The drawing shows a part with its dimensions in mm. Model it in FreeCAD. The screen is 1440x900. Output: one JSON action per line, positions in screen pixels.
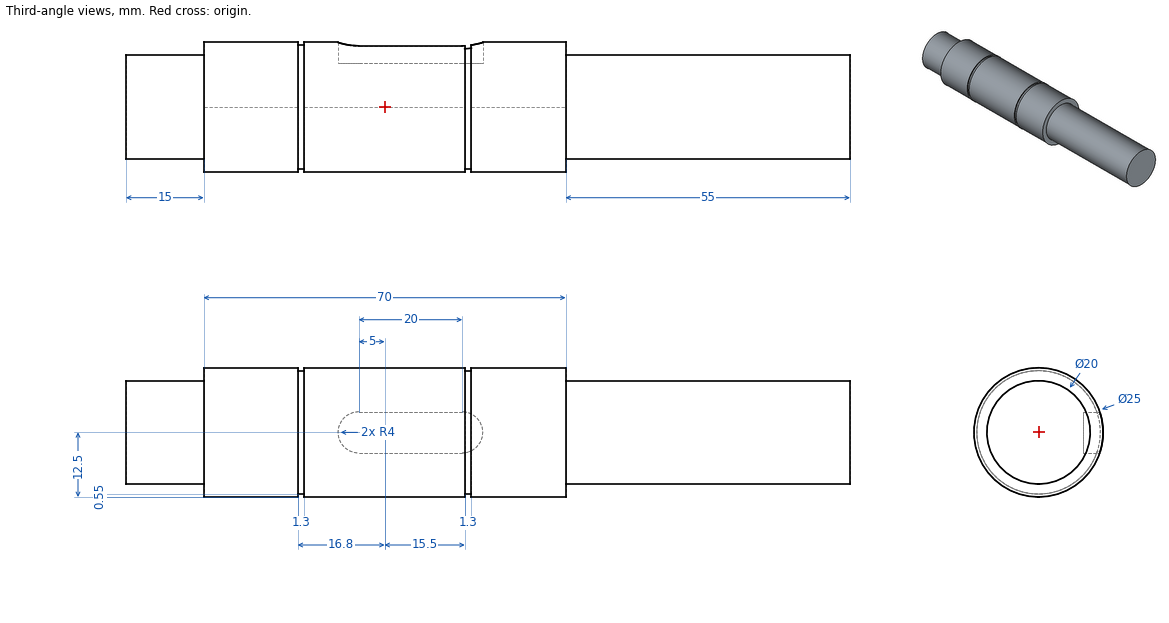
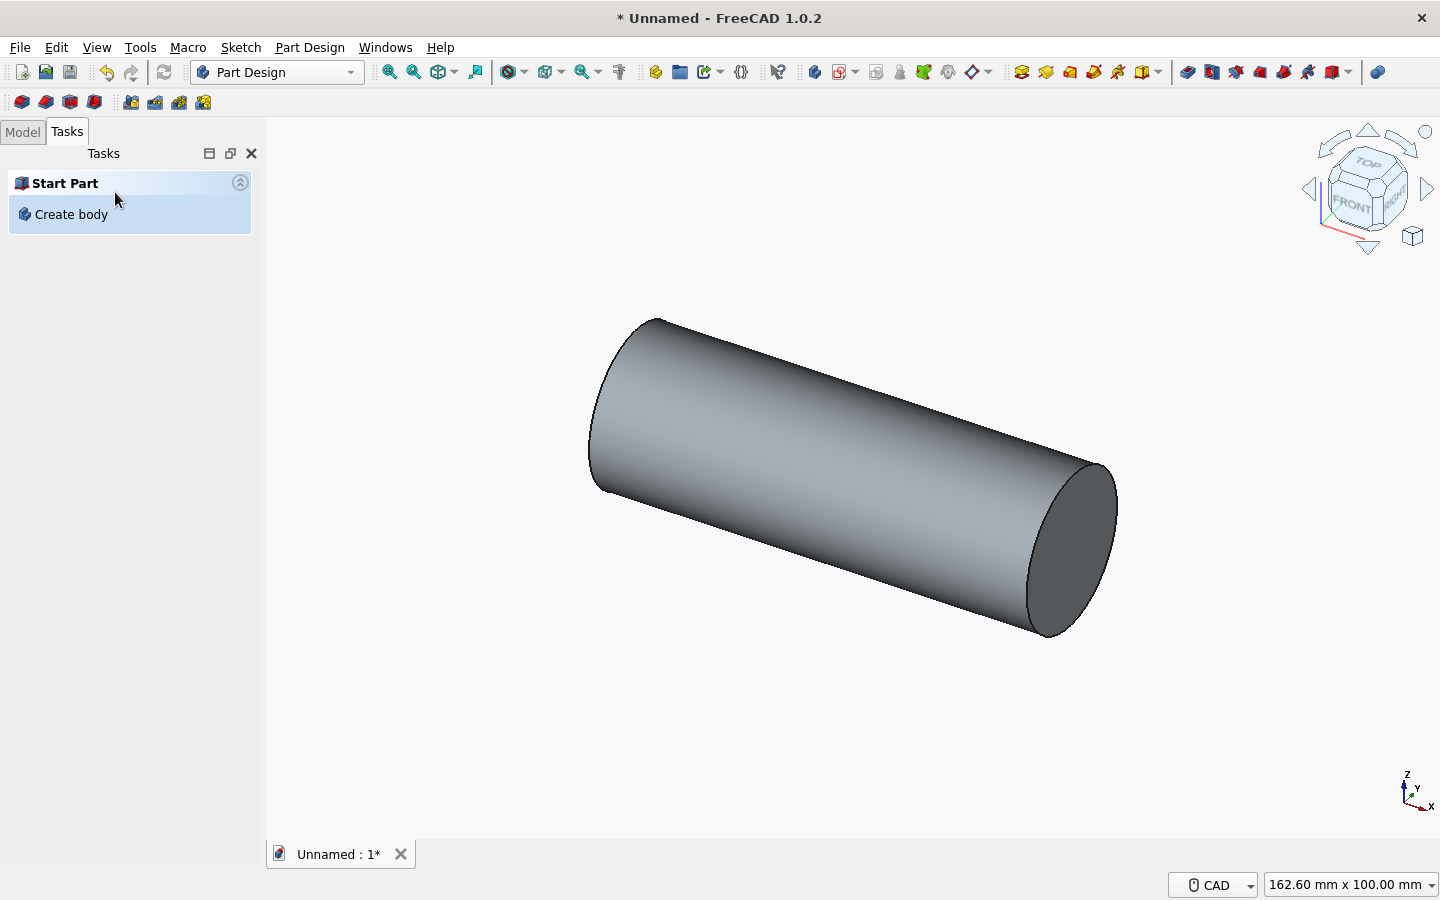
{"action": "left_click", "coordinate": [1072, 549]}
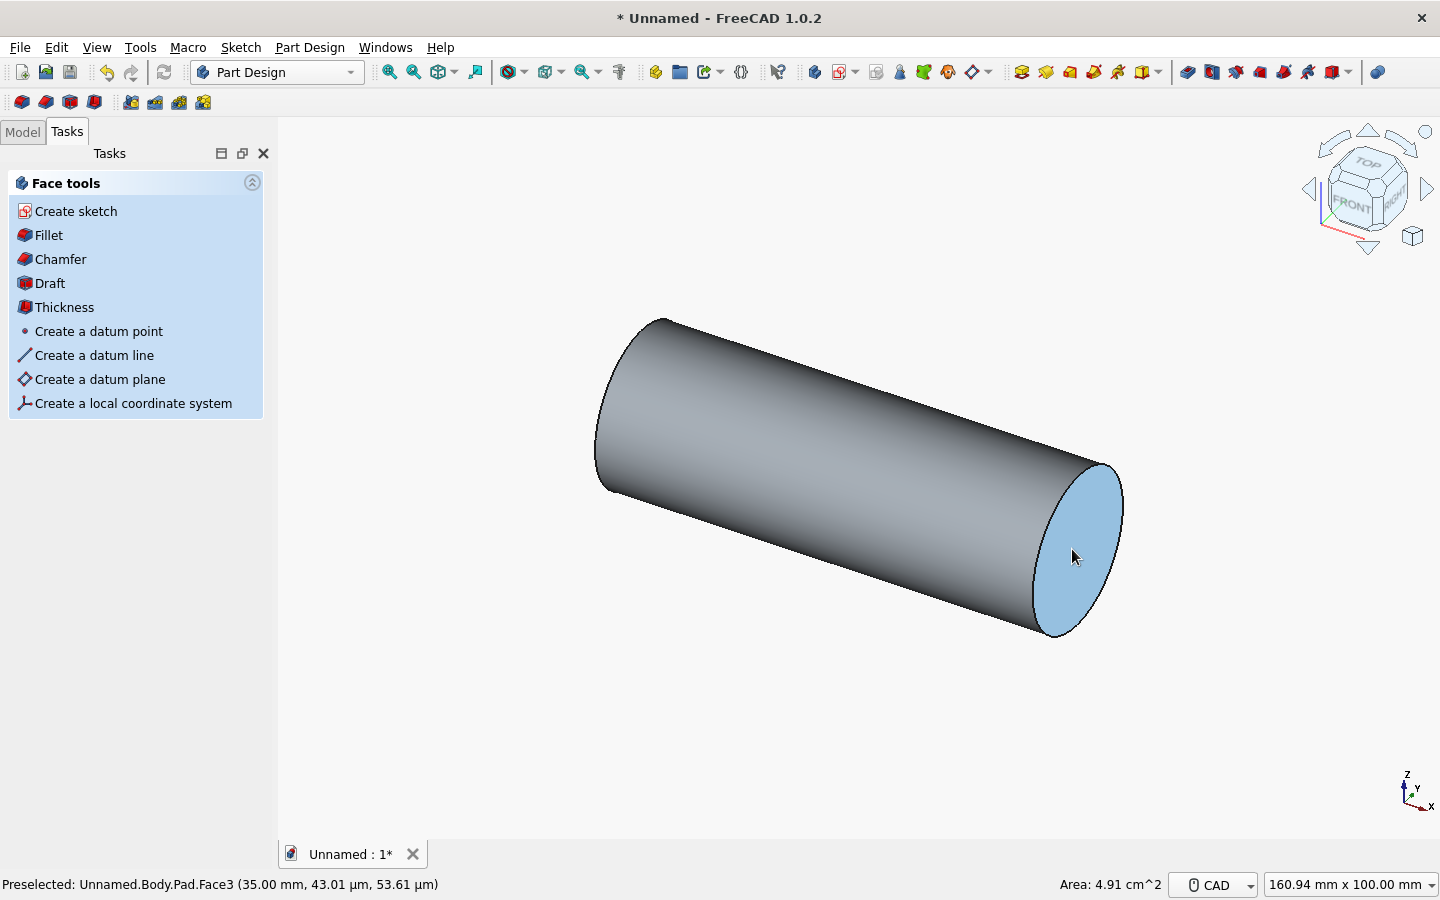
{"action": "left_click", "coordinate": [840, 72]}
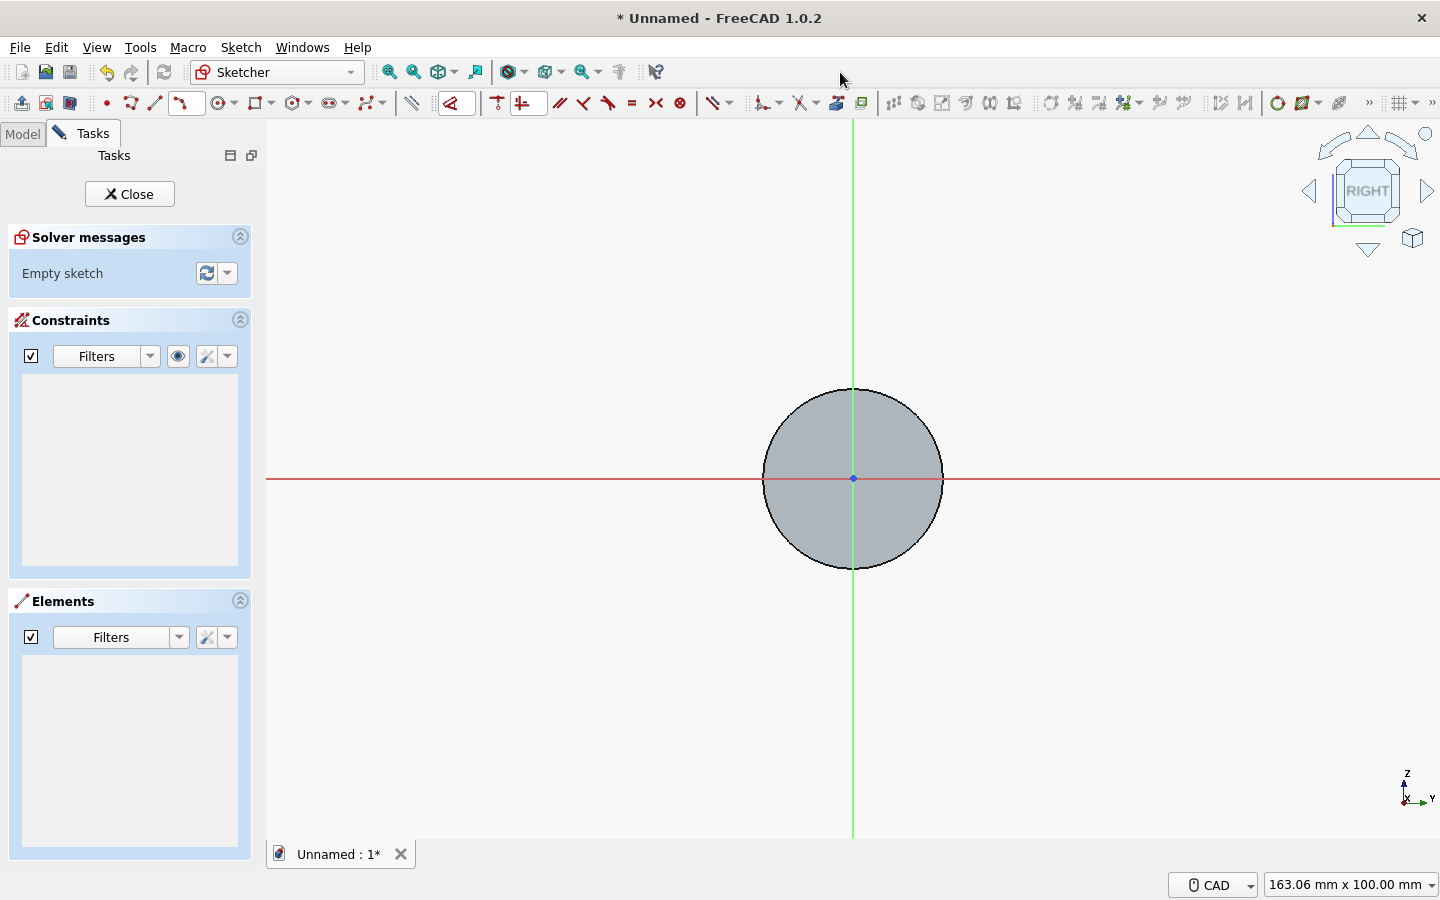
{"action": "scroll", "coordinate": [883, 479], "scroll_direction": "up", "scroll_amount": 6}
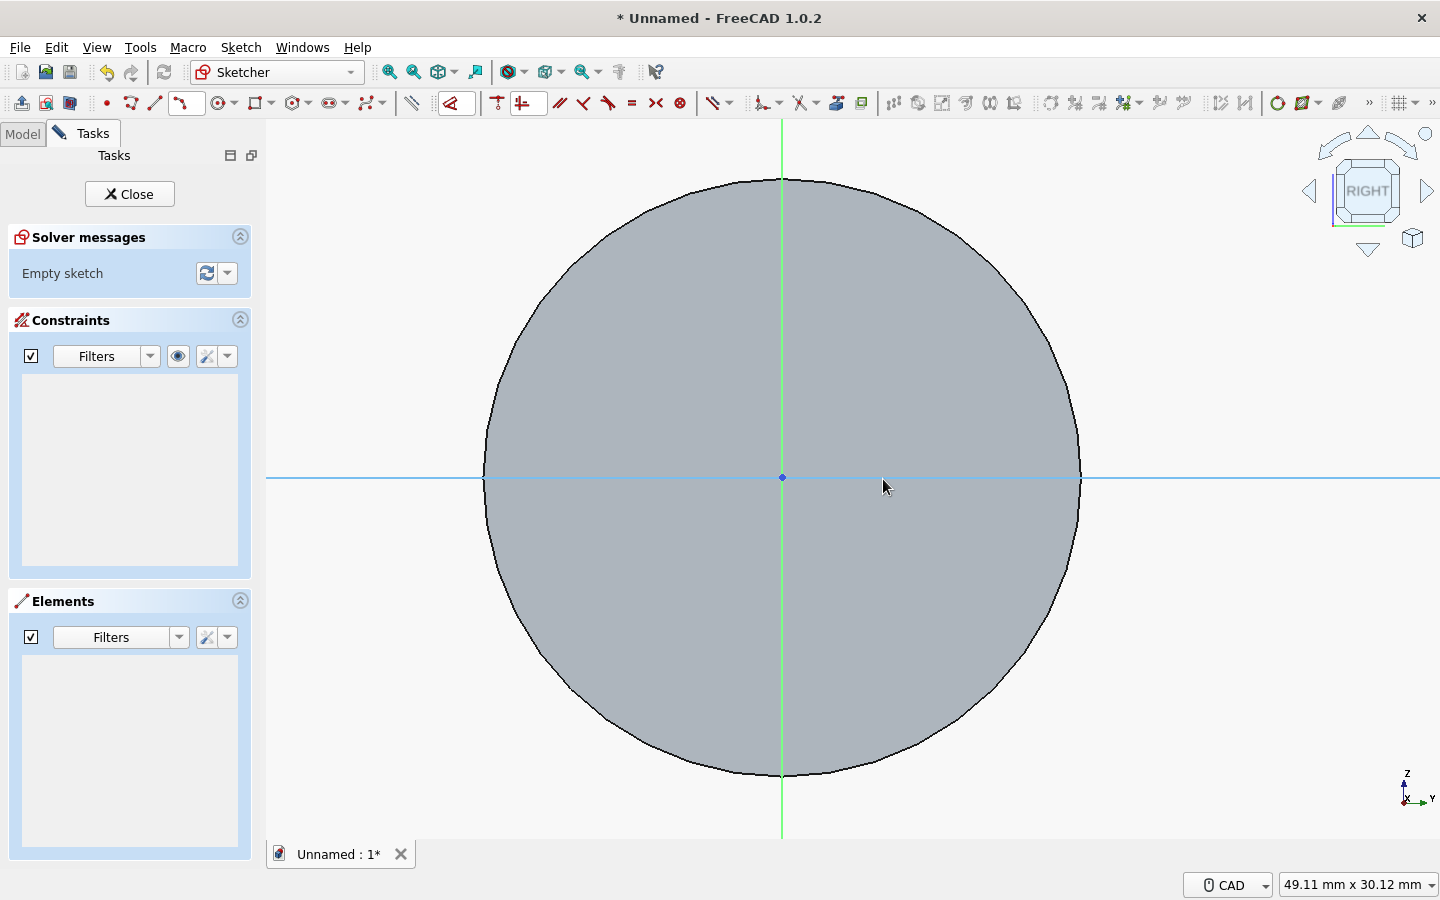
{"action": "left_click", "coordinate": [218, 104]}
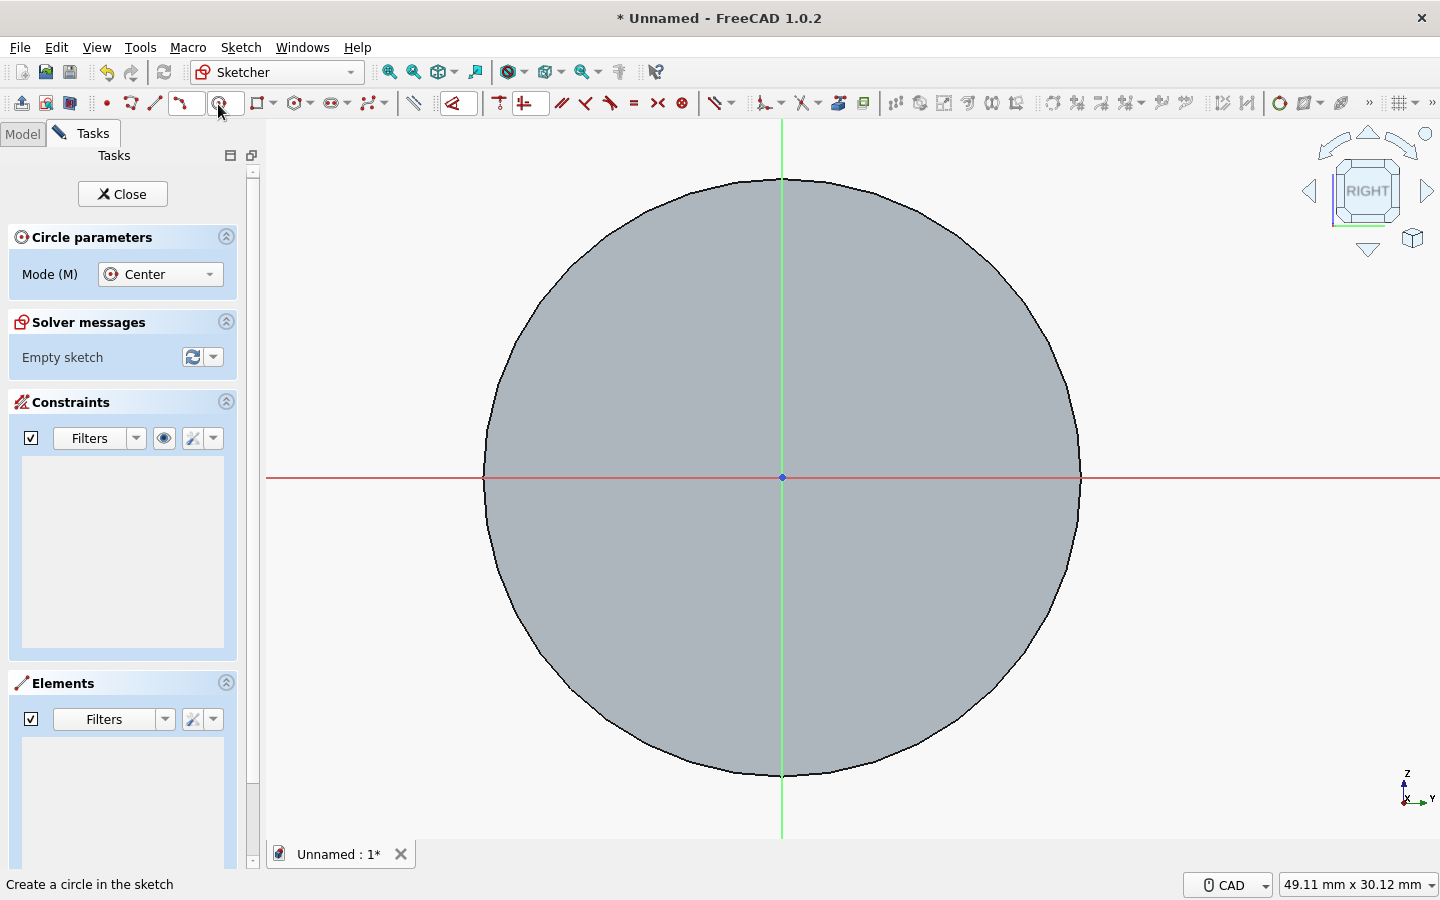
{"action": "left_click", "coordinate": [782, 478]}
{"action": "left_click", "coordinate": [951, 309]}
{"action": "key", "text": "Escape"}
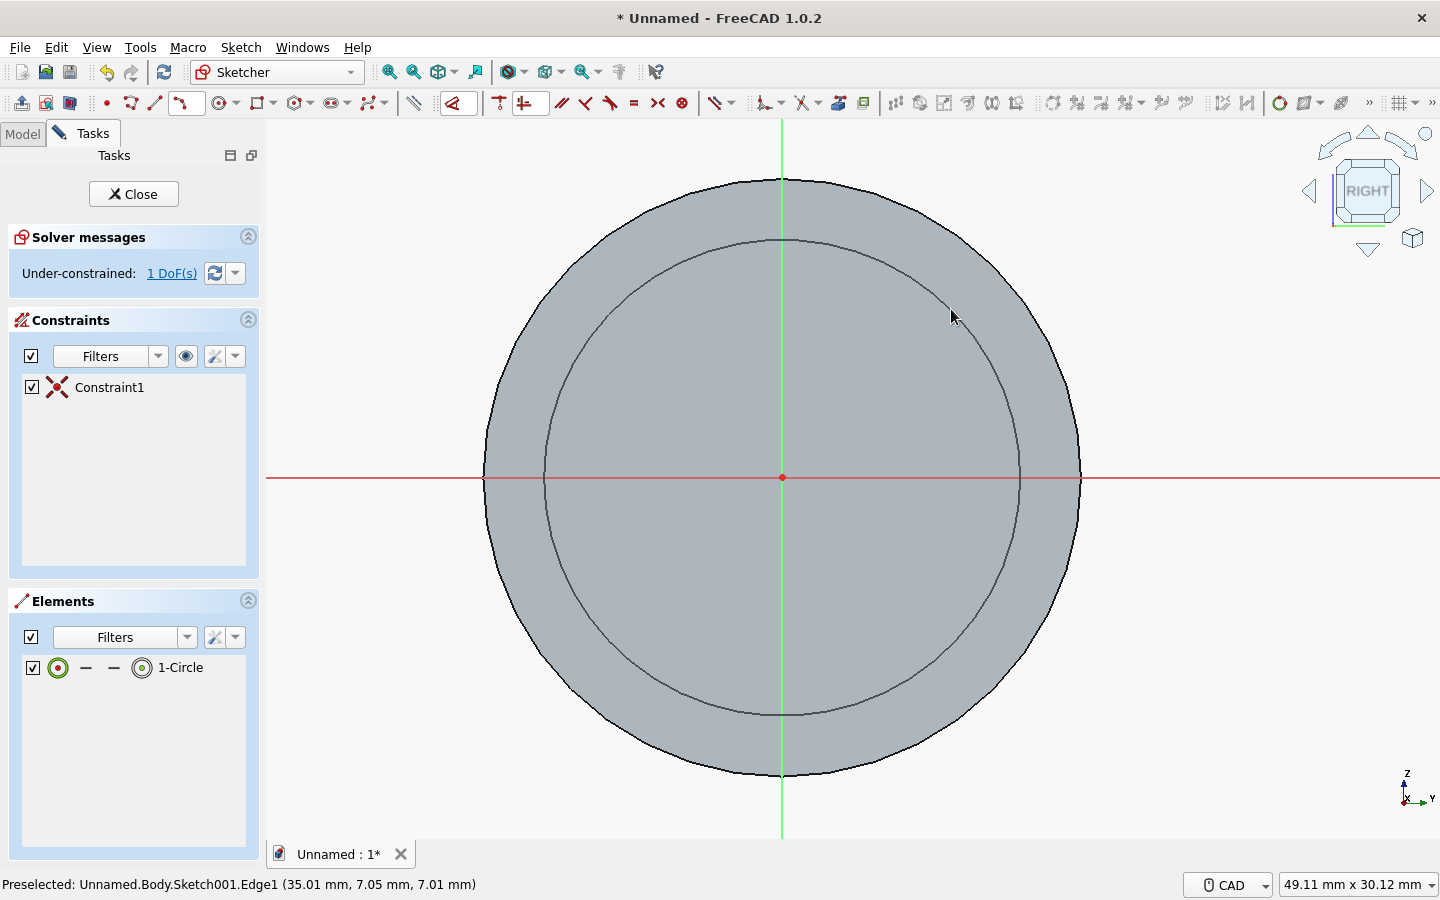
{"action": "left_click", "coordinate": [950, 309]}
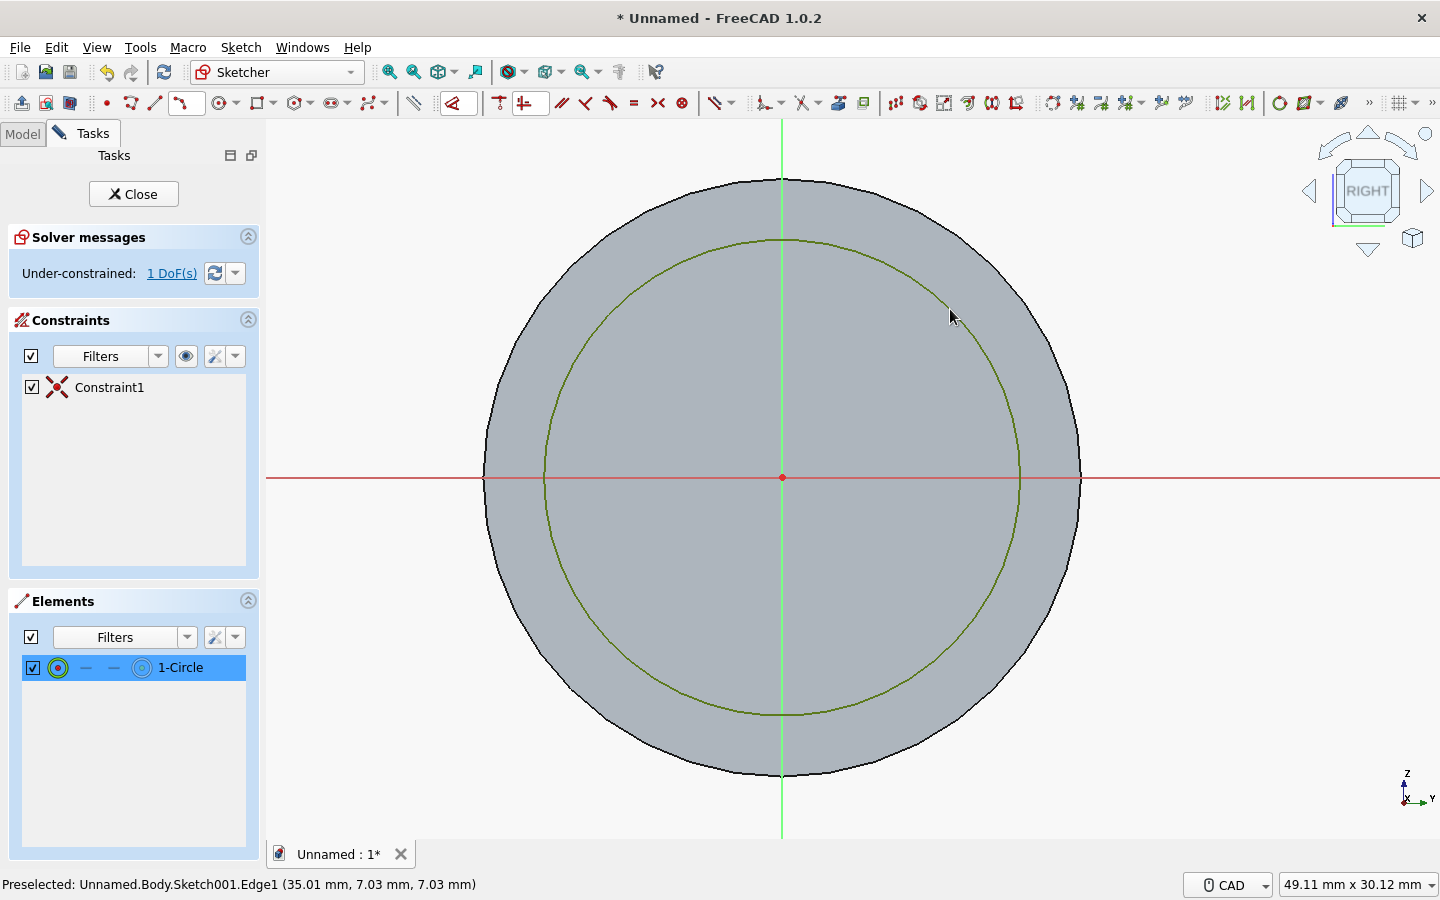
{"action": "left_click", "coordinate": [472, 104]}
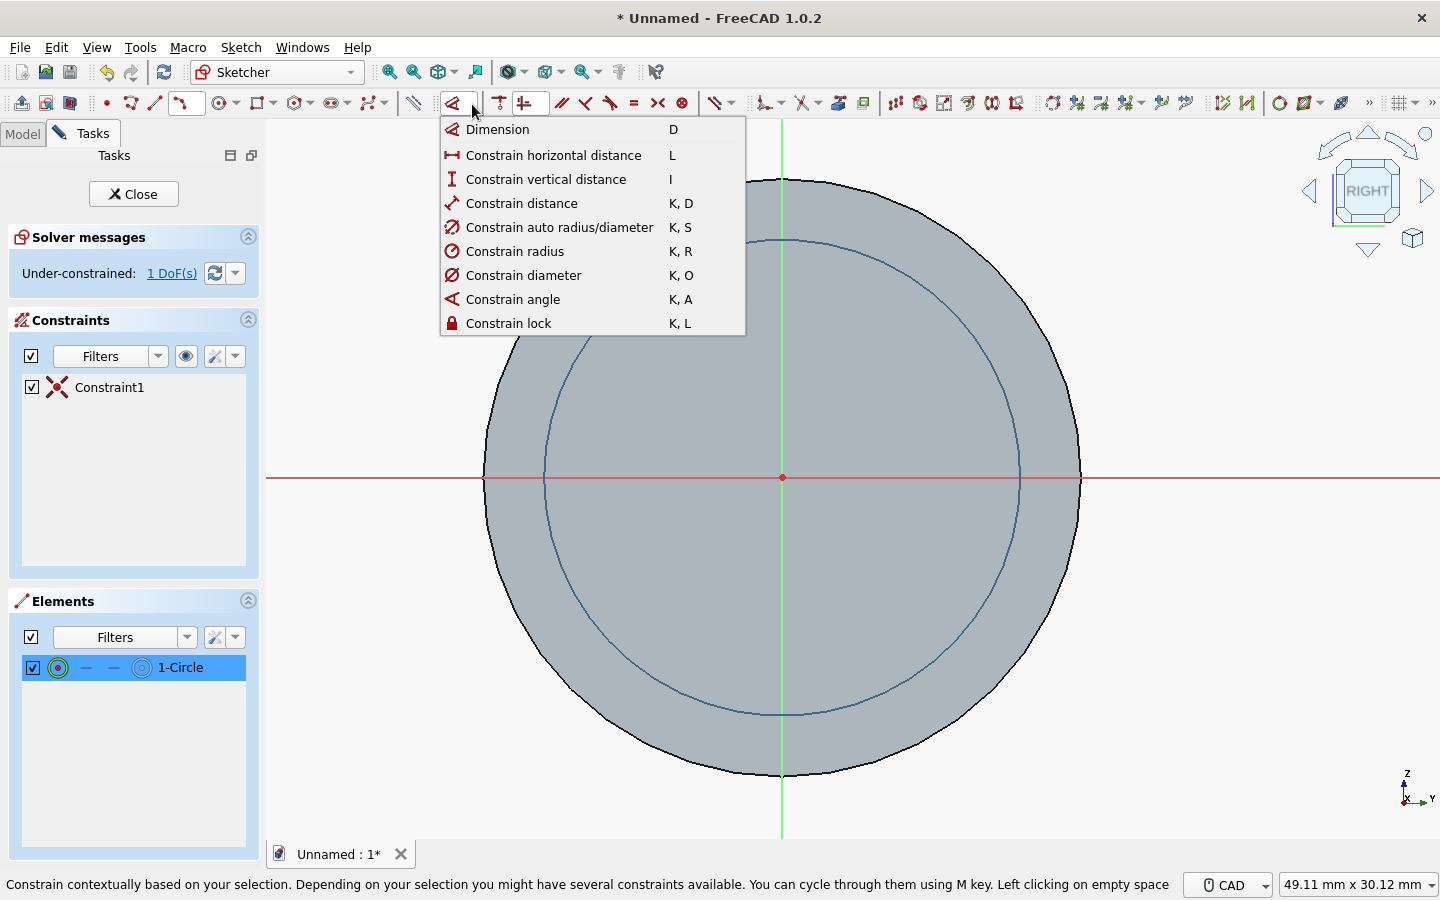
{"action": "left_click", "coordinate": [593, 275]}